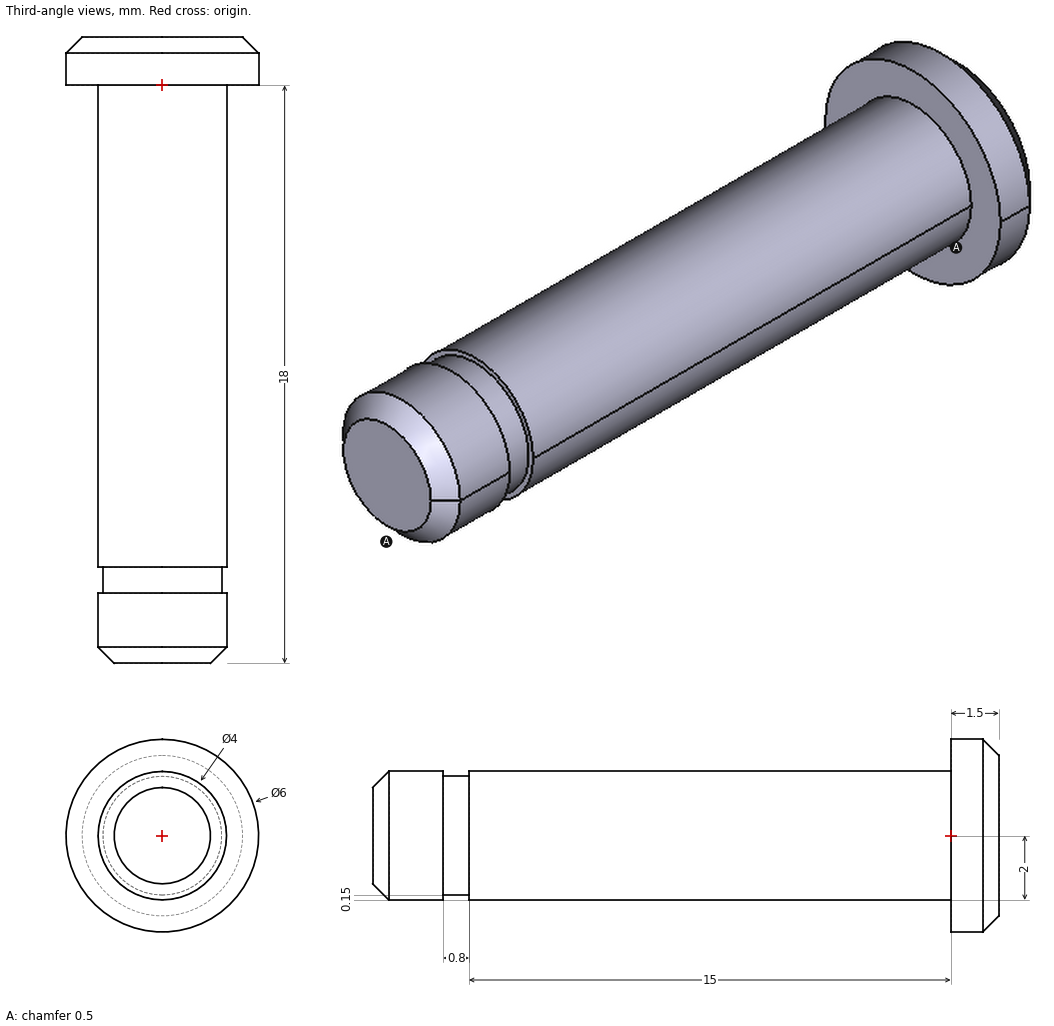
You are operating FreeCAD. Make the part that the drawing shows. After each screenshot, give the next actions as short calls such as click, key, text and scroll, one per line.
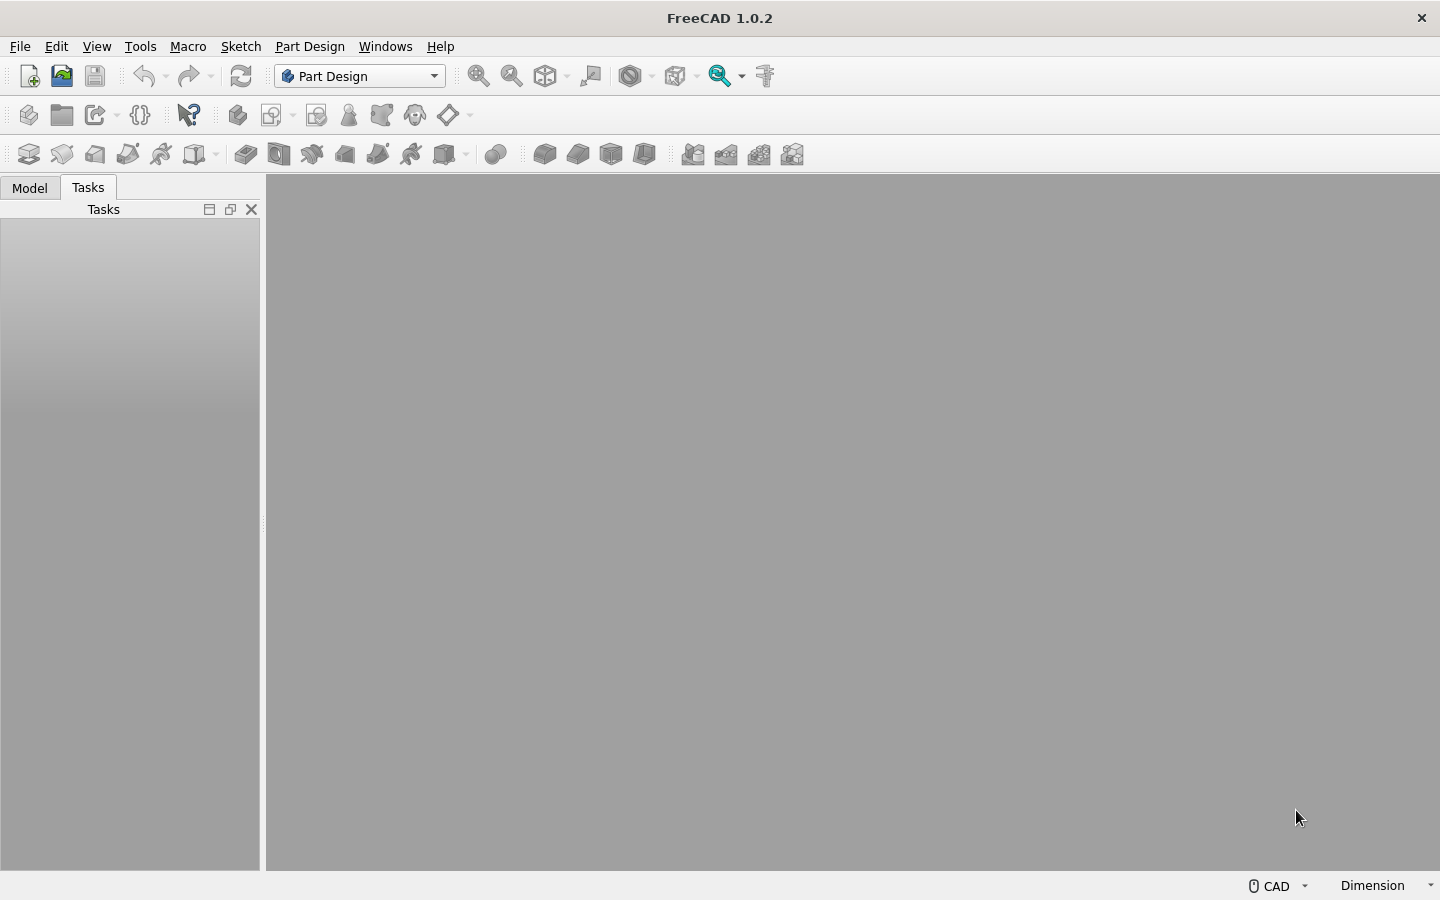
key(ctrl+n)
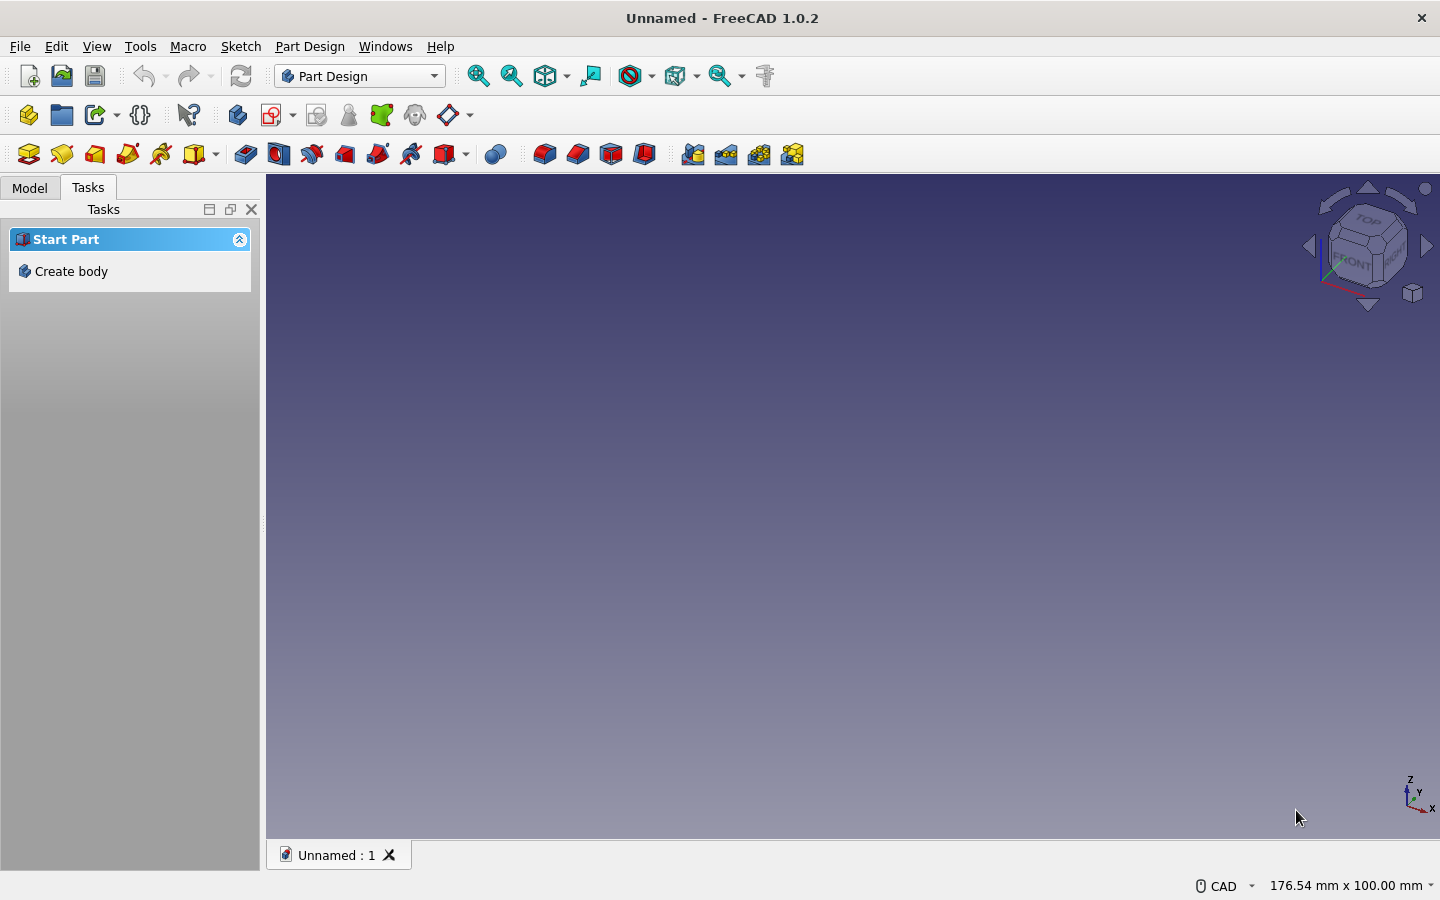
click(270, 116)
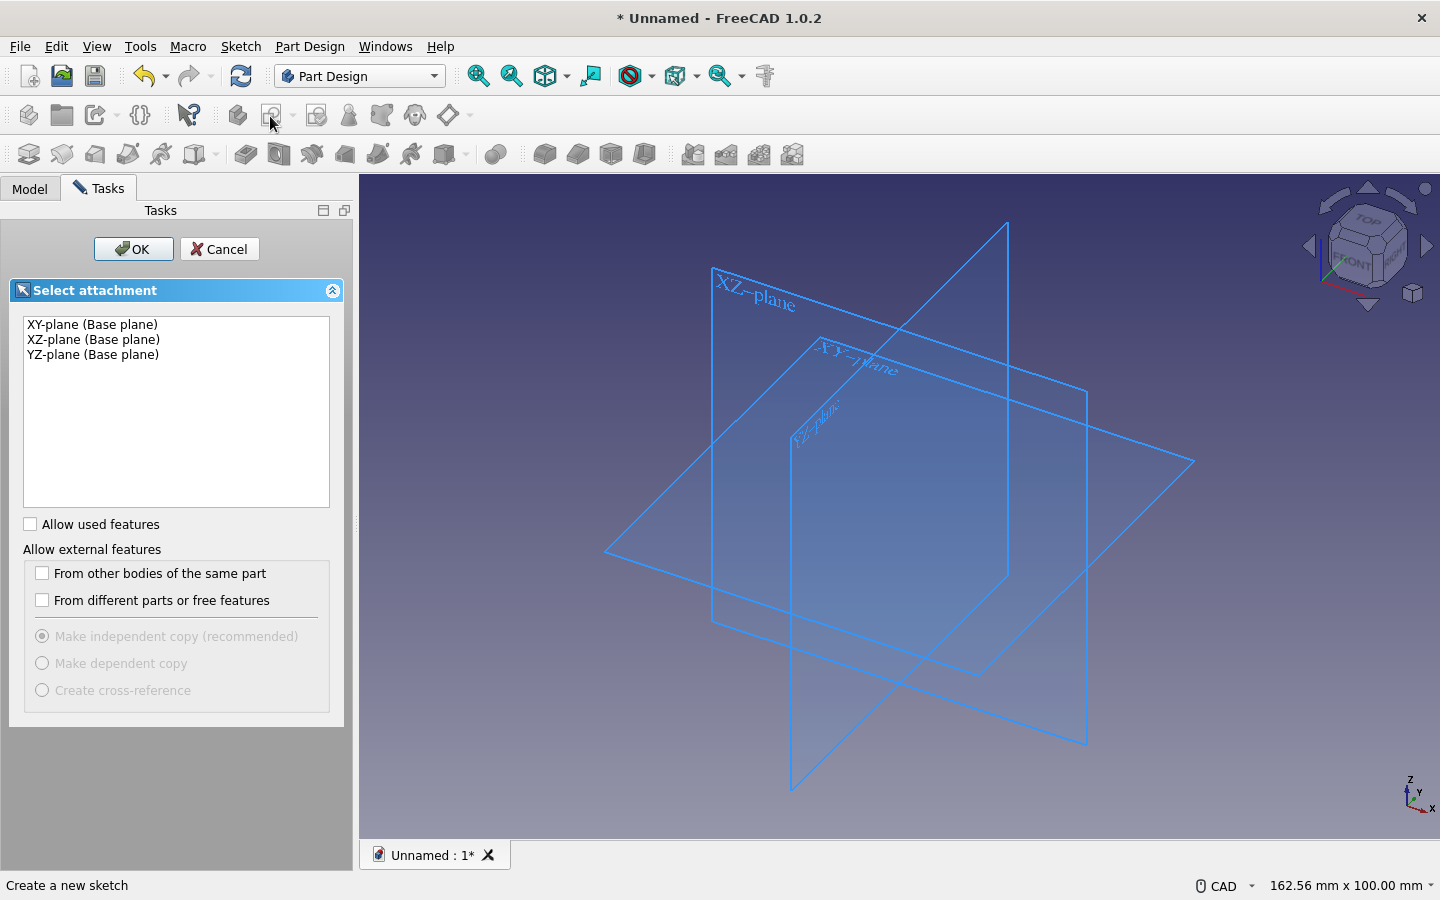
click(84, 340)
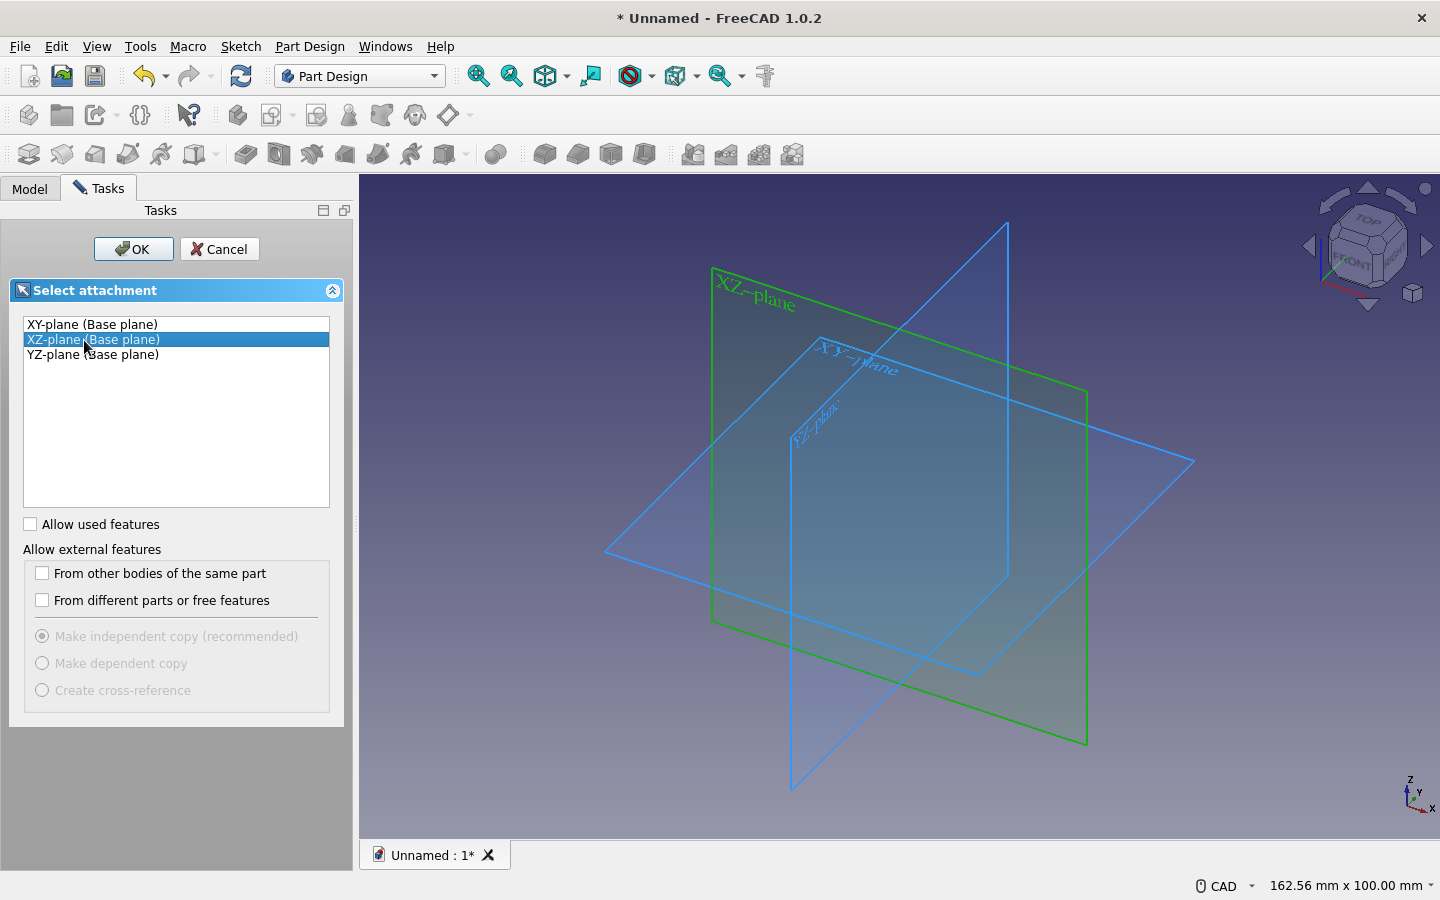
click(134, 249)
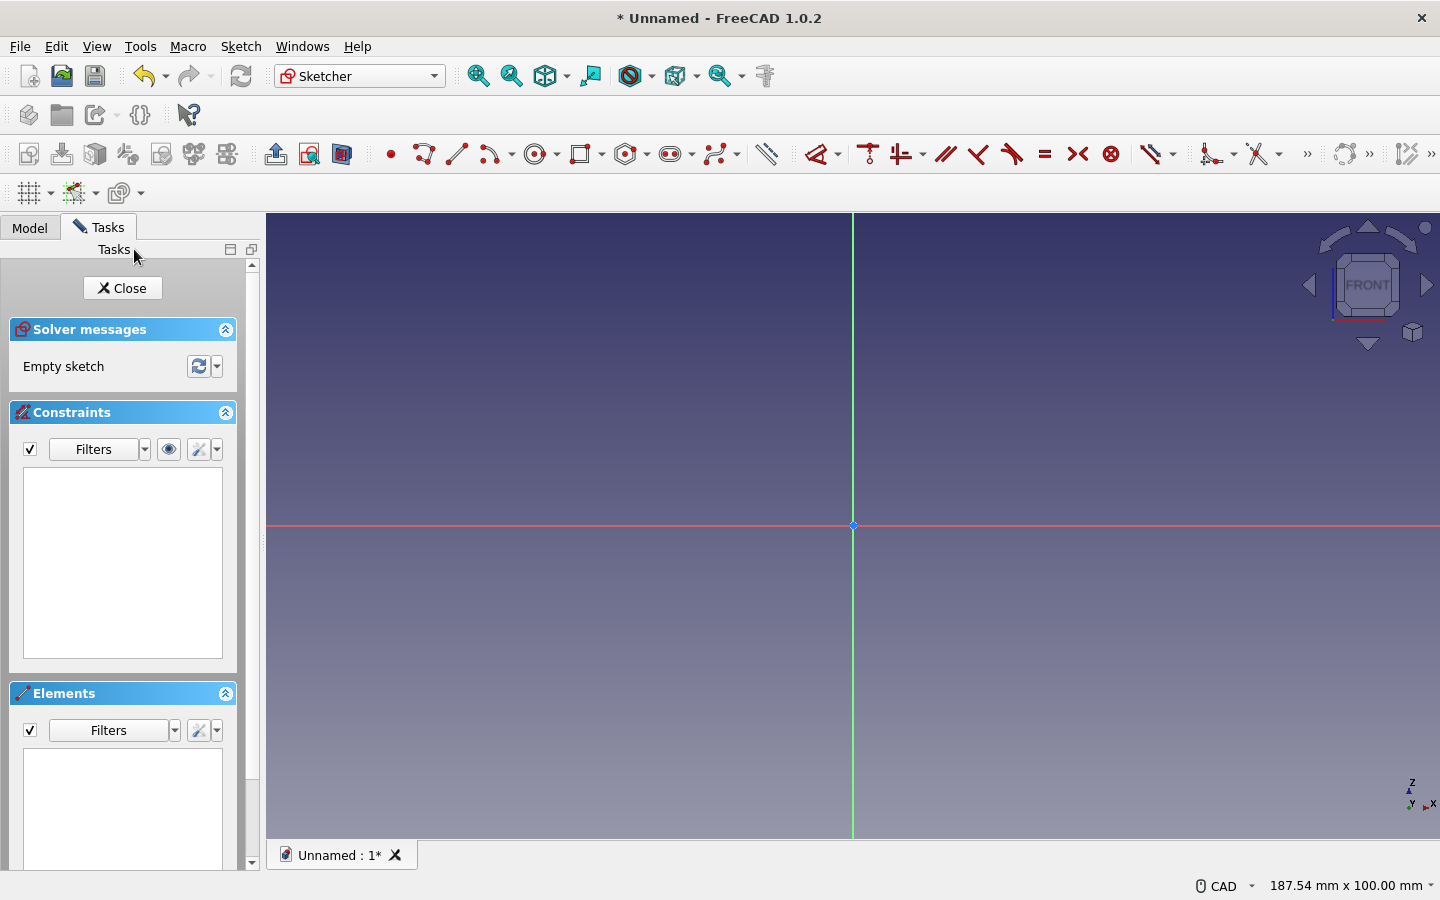
scroll(860, 526, up, 12)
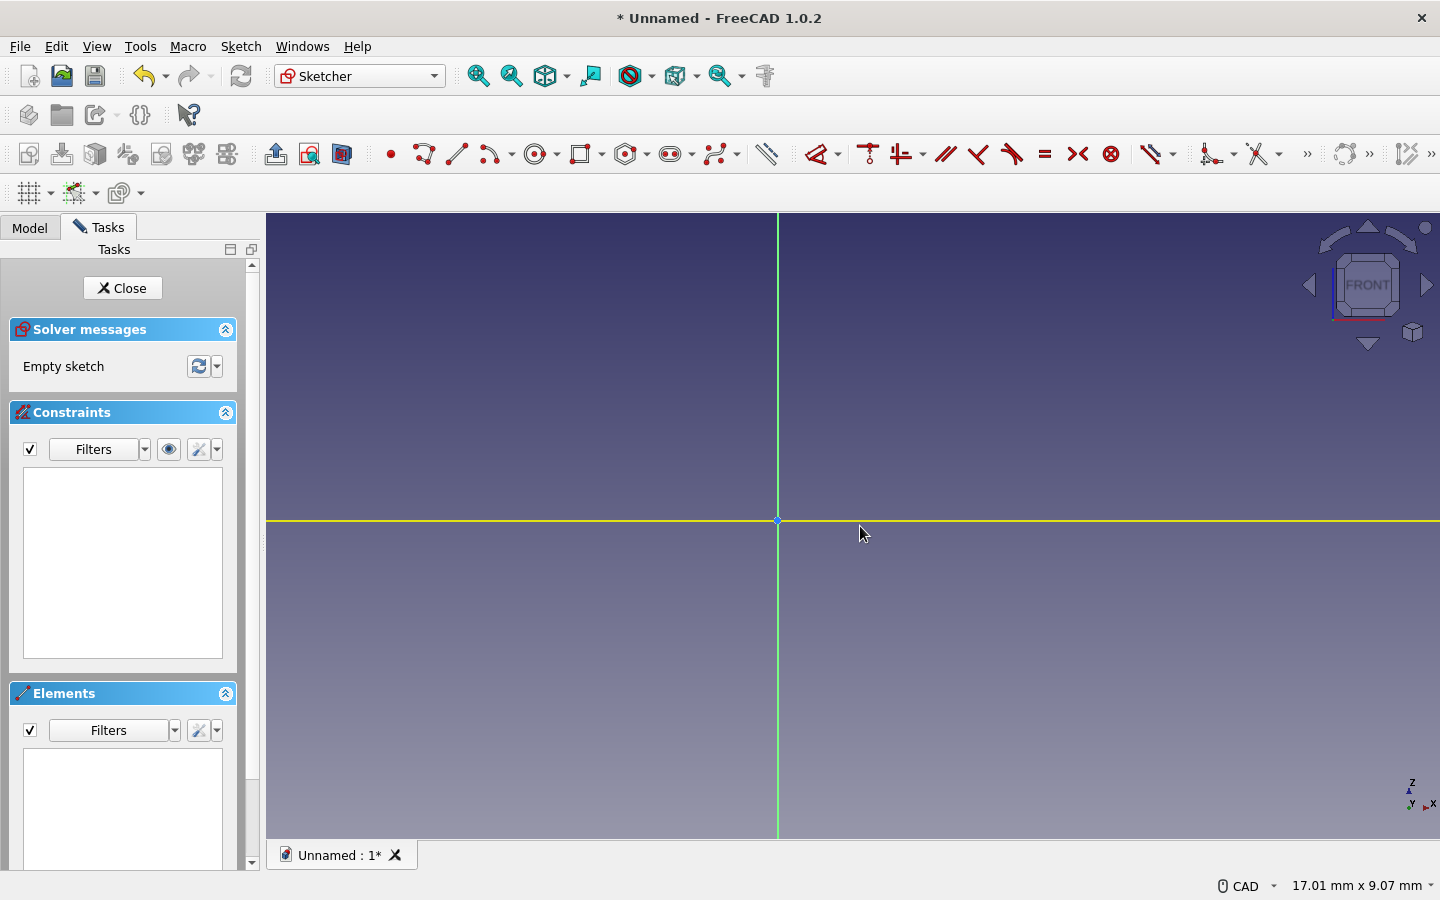
key(g)
key(c)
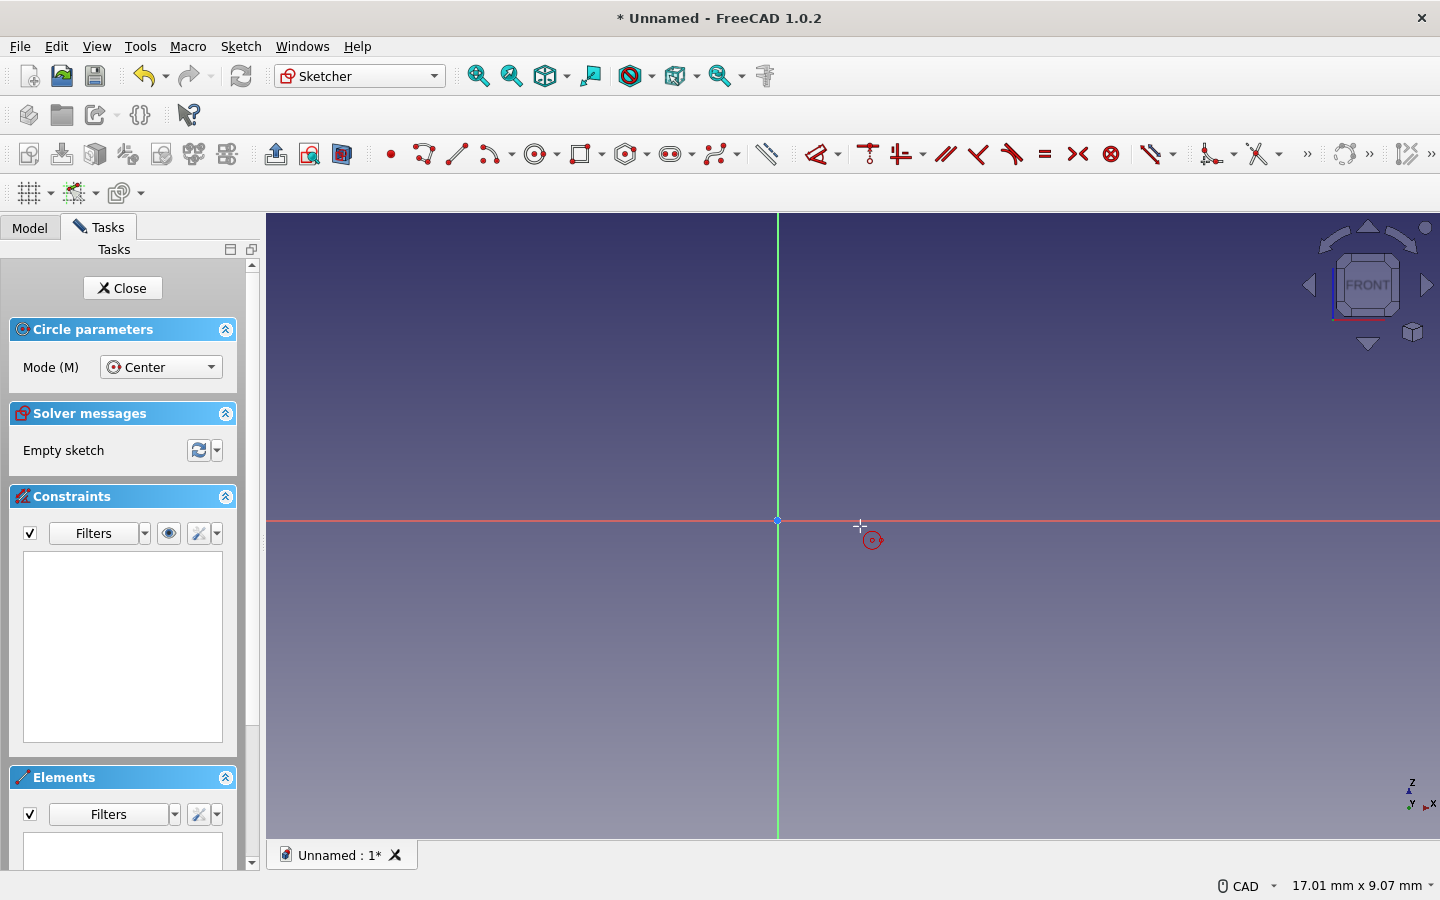
click(778, 521)
move(924, 375)